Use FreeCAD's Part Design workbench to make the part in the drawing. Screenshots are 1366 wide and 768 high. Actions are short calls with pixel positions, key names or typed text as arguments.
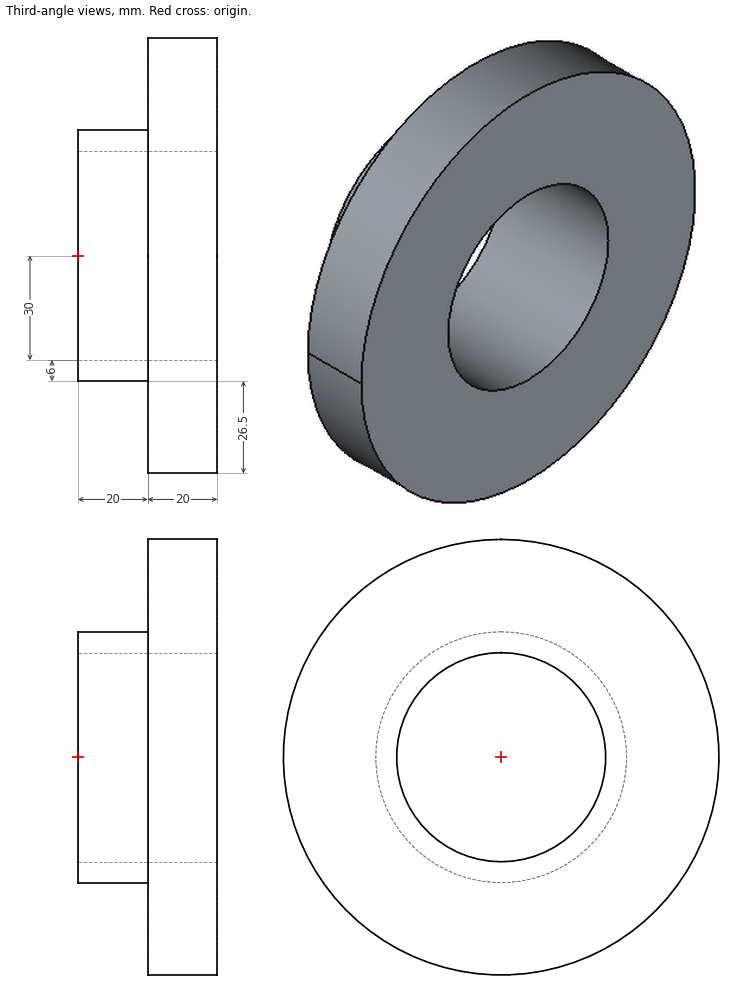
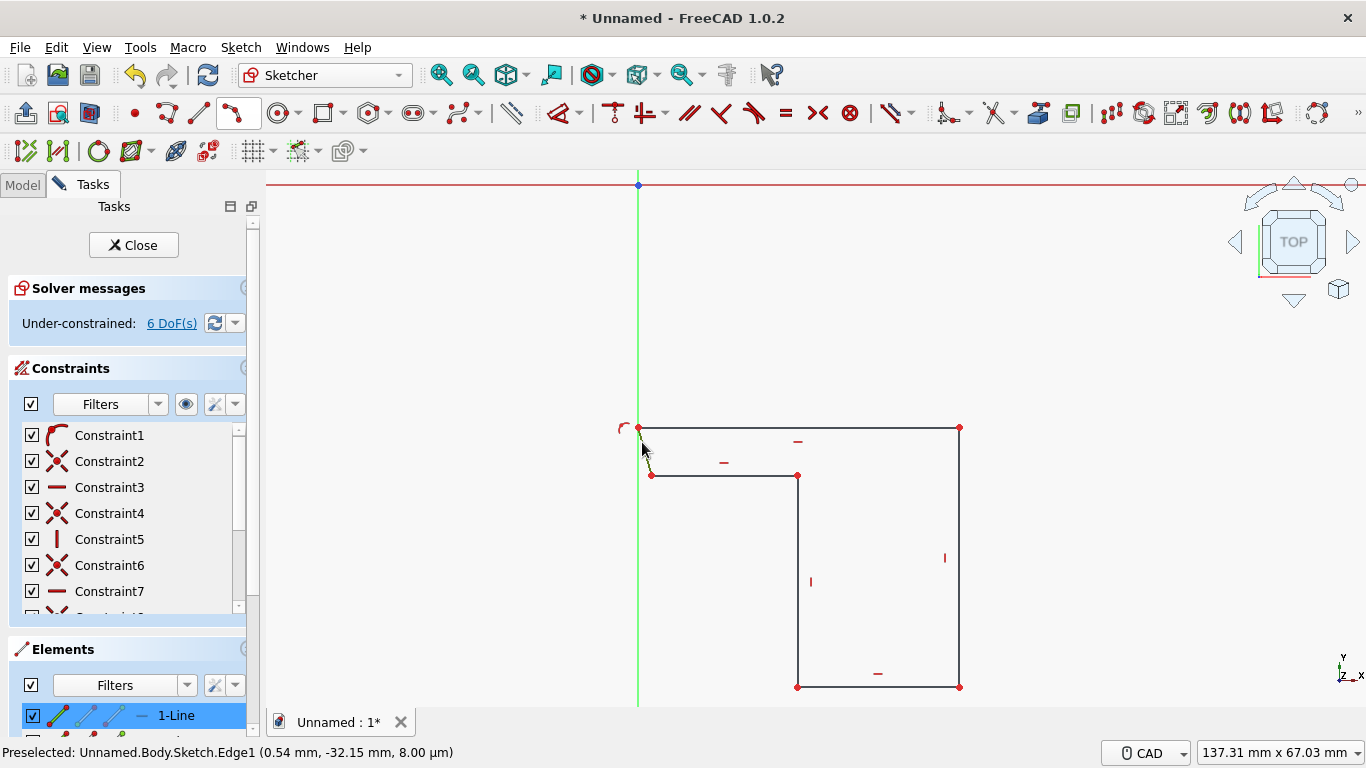
click(668, 114)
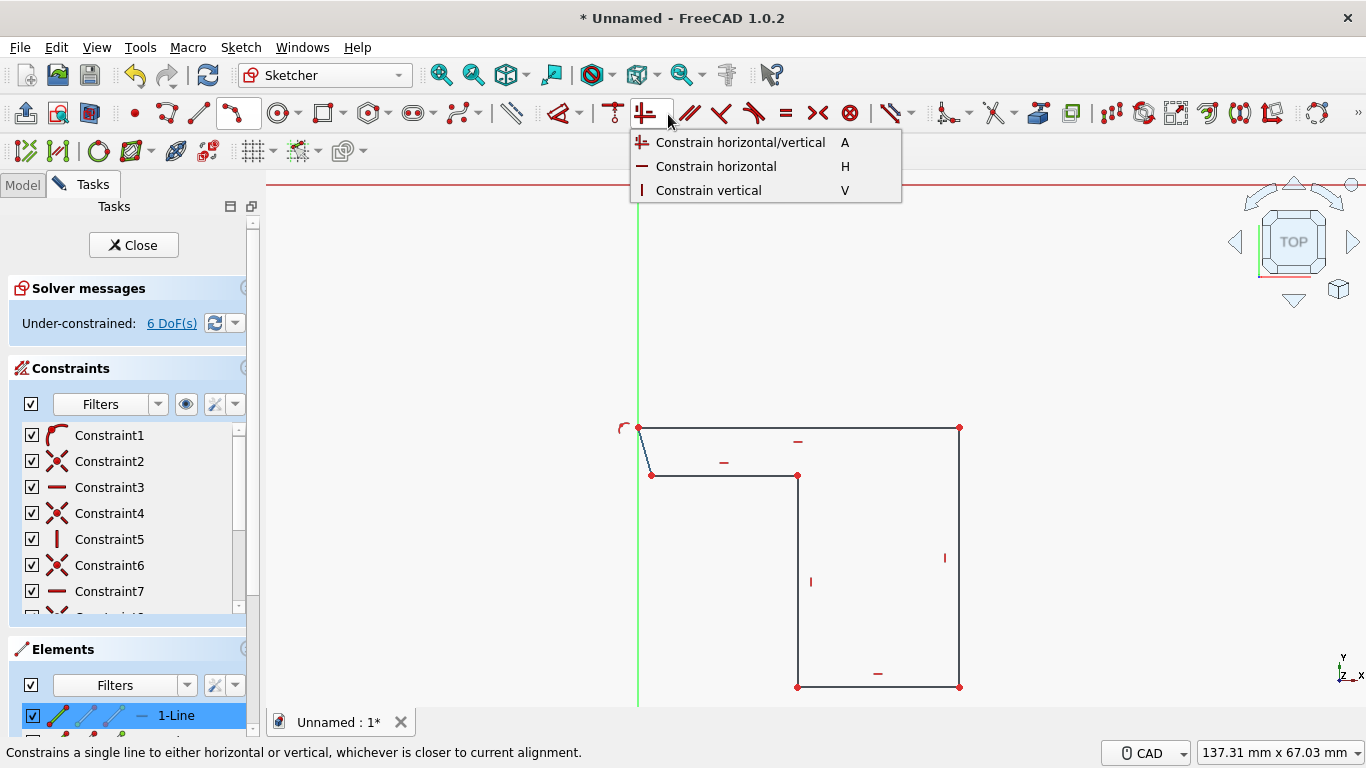
click(766, 190)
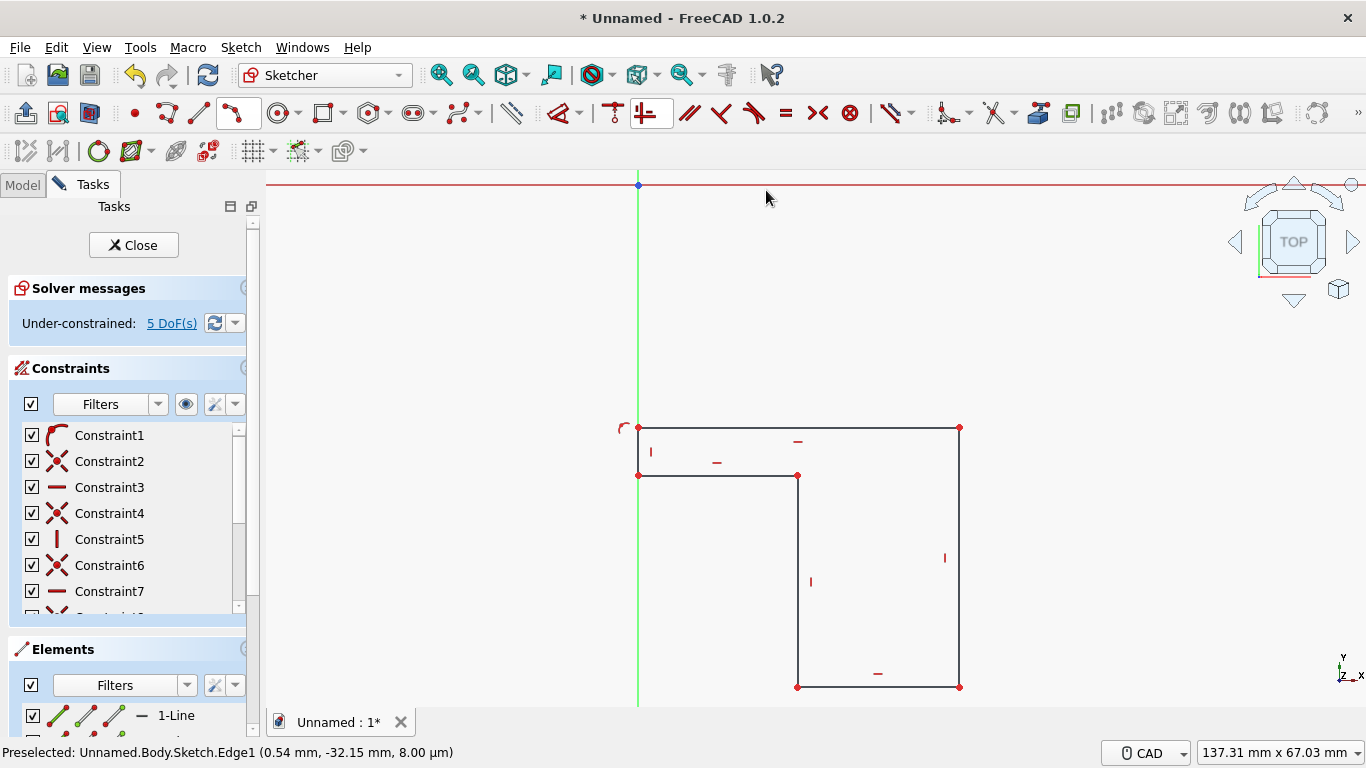
click(638, 442)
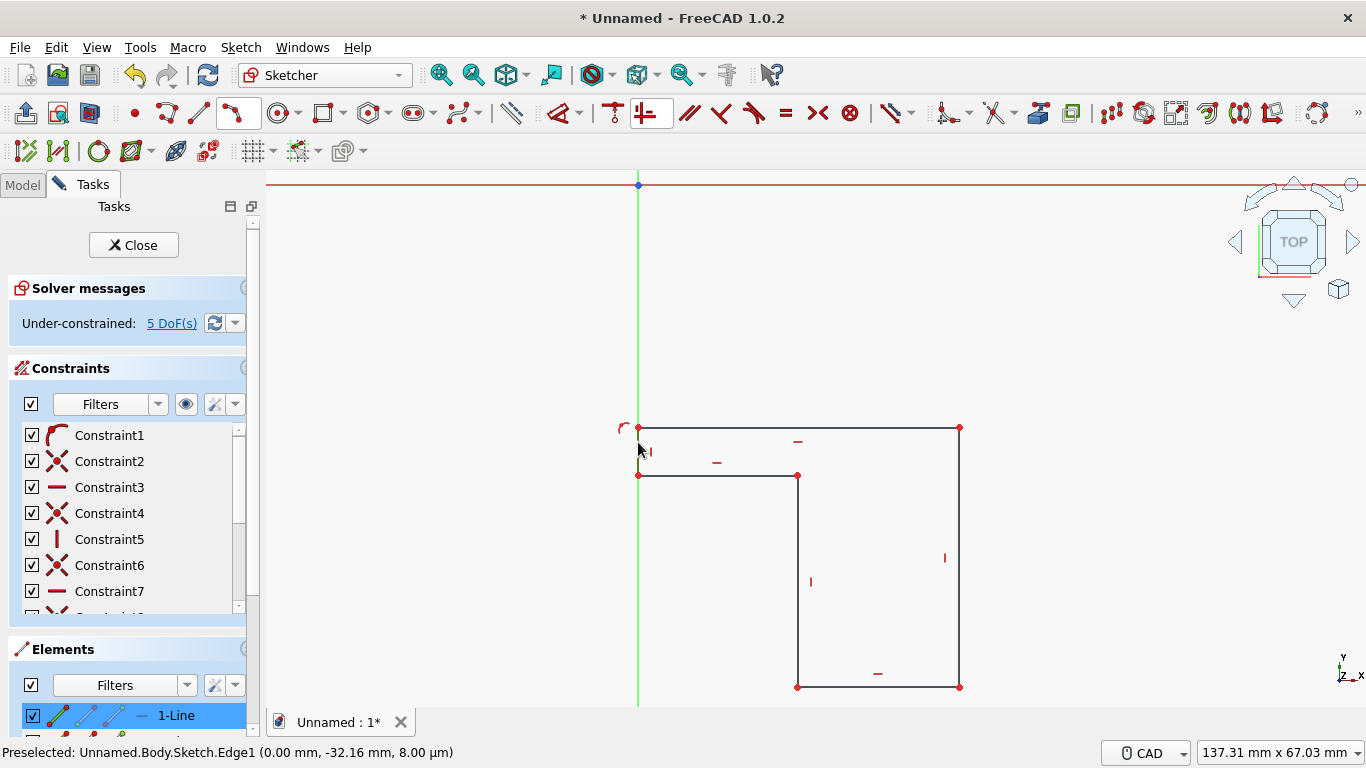
key(i)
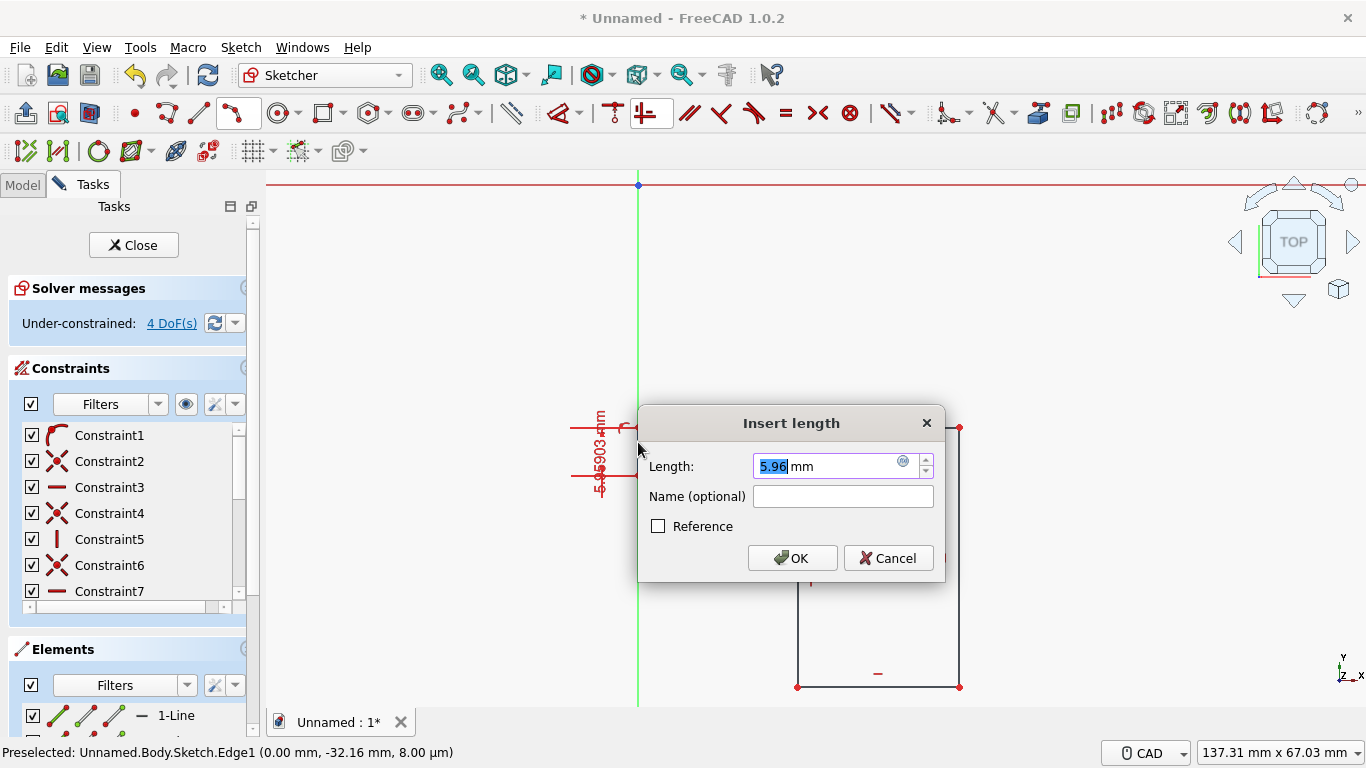
text(6)
key(Return)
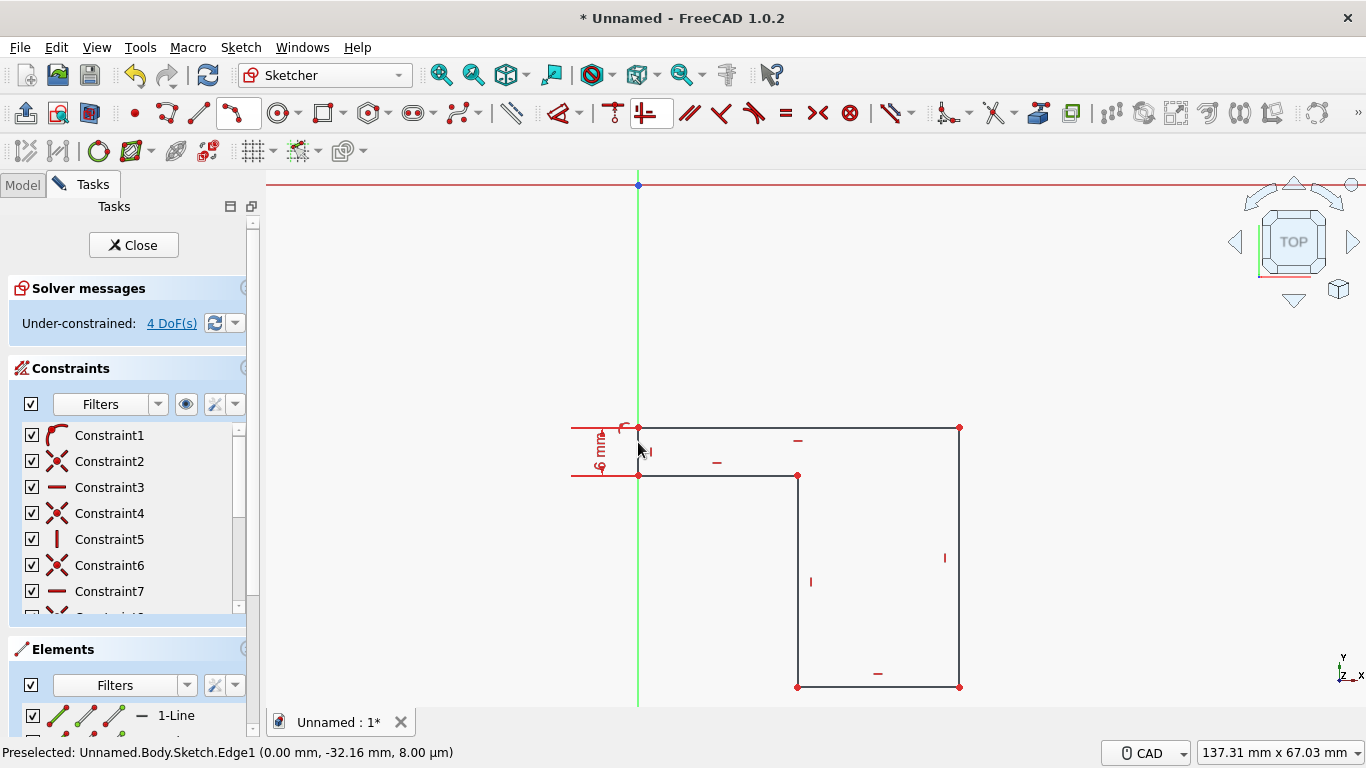
click(686, 476)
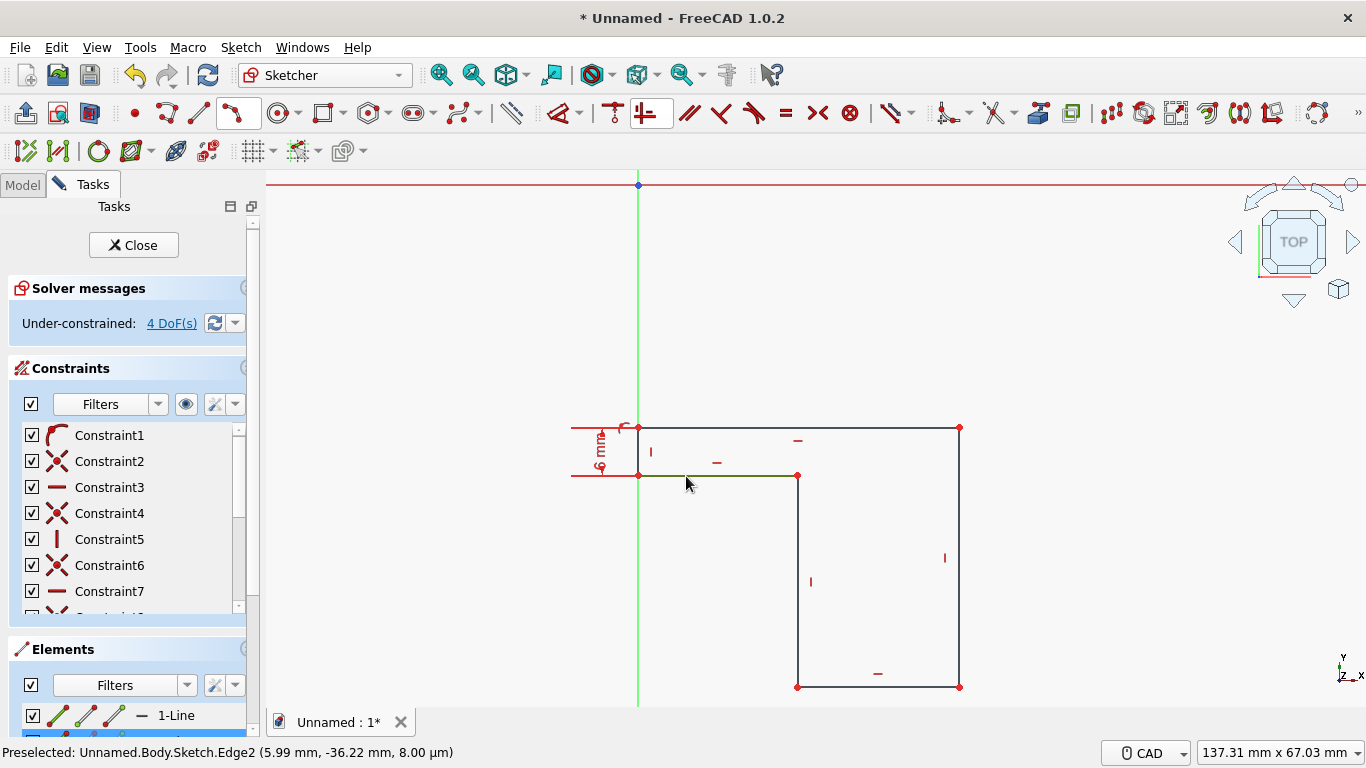
click(582, 114)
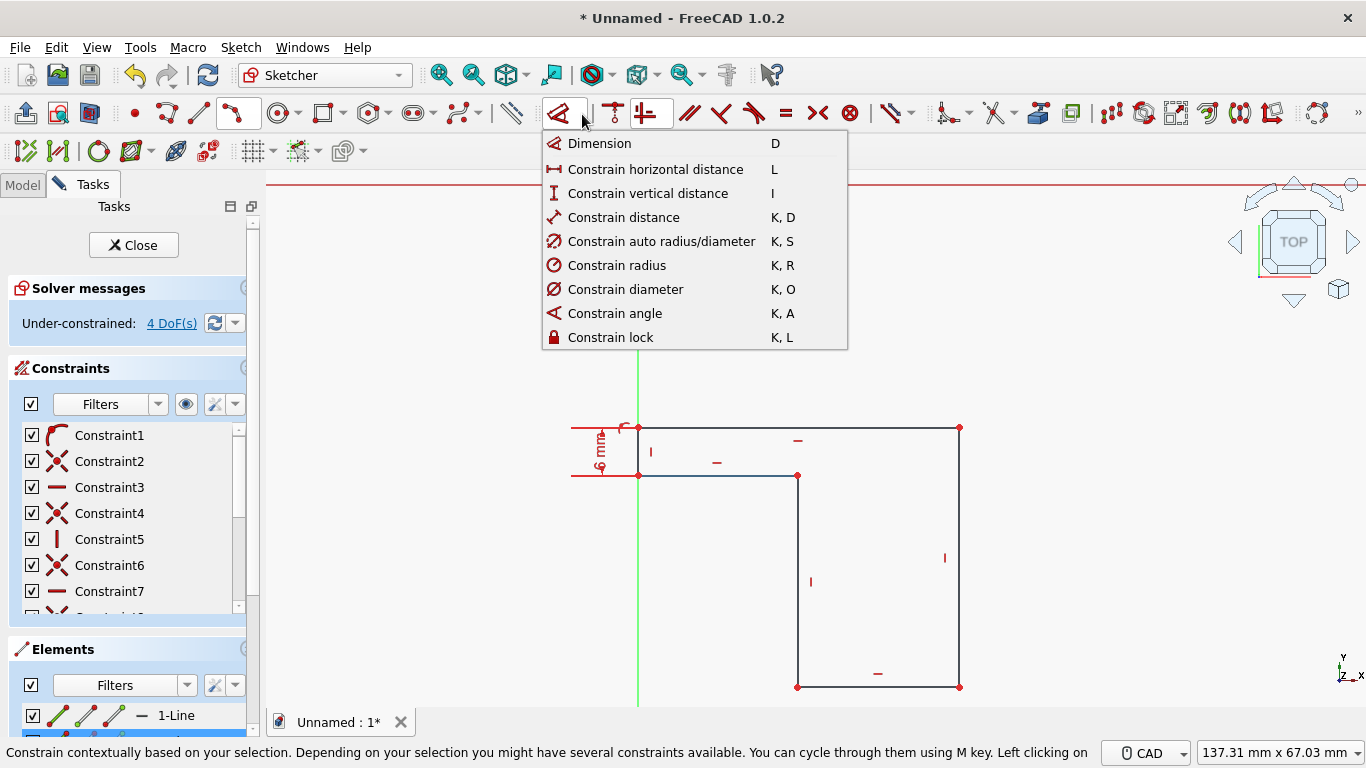
click(695, 169)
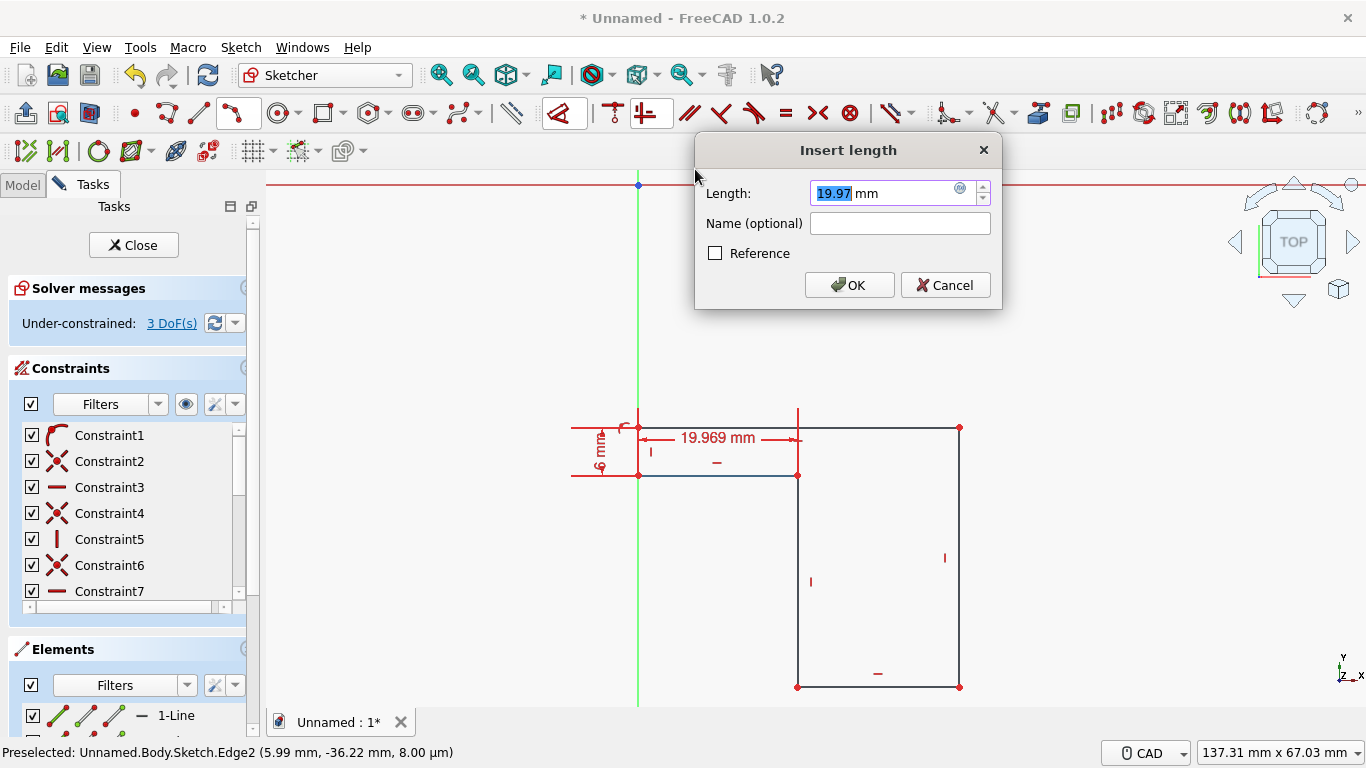
text(20)
key(Return)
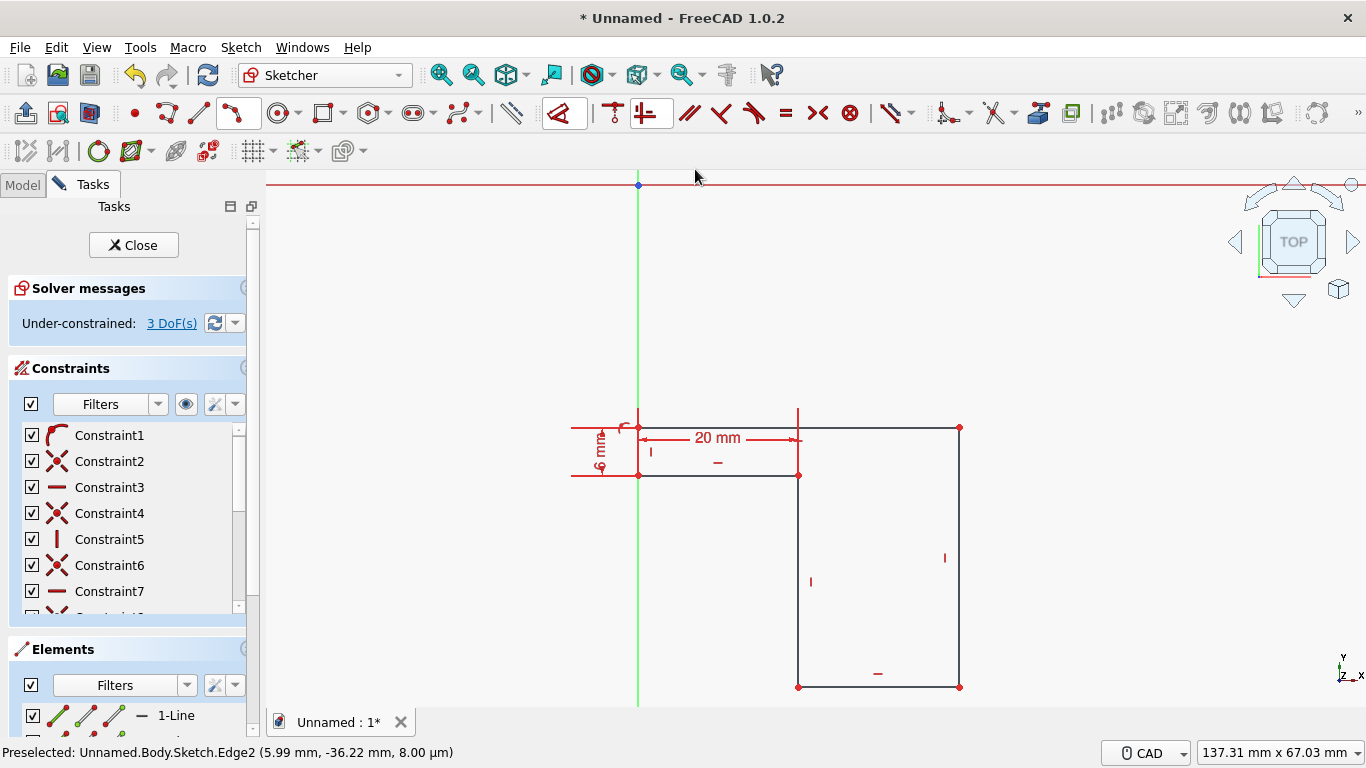
scroll(644, 444, down, 2)